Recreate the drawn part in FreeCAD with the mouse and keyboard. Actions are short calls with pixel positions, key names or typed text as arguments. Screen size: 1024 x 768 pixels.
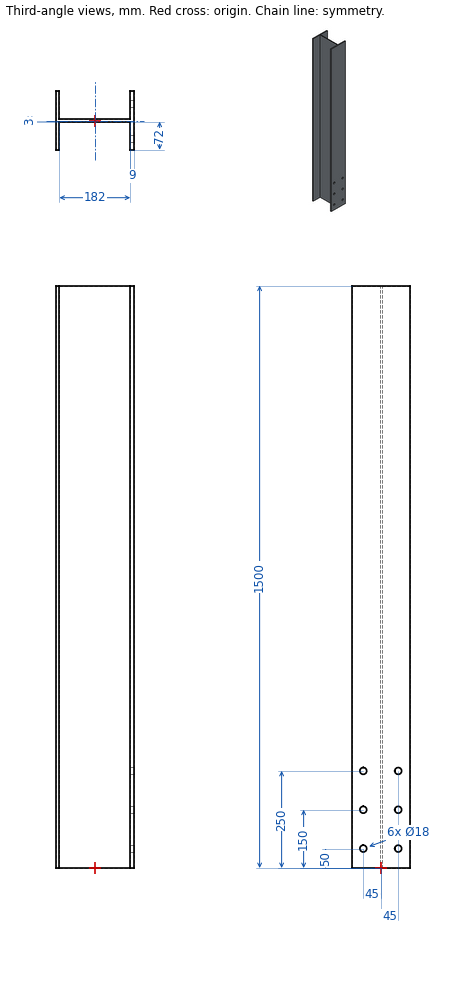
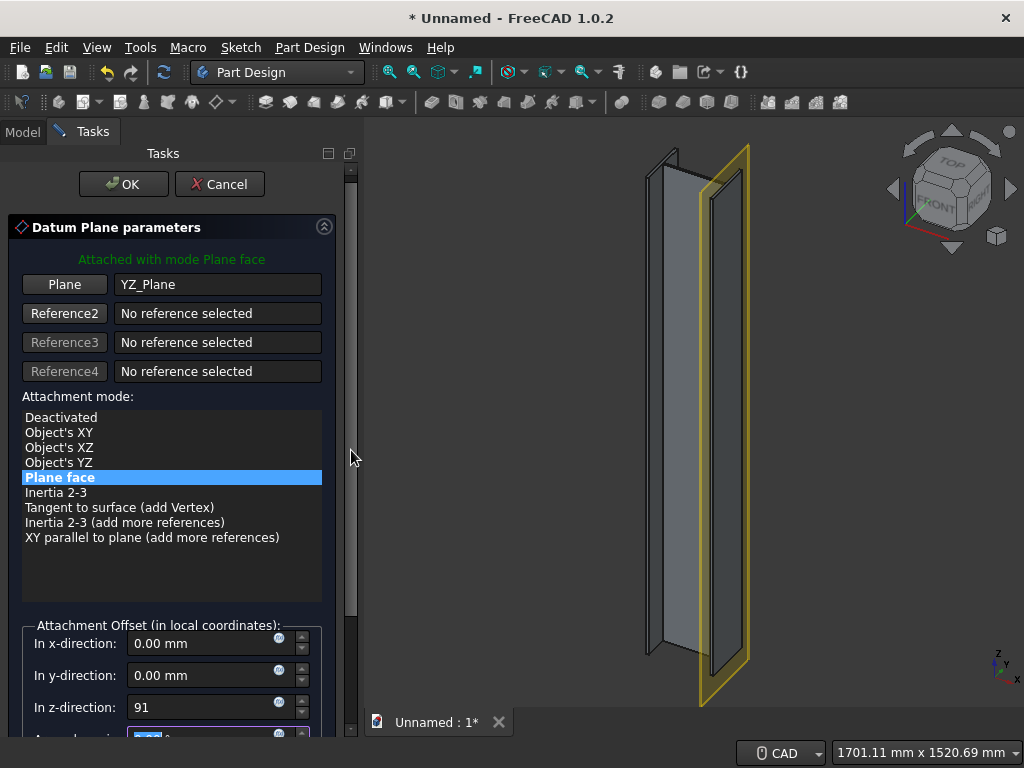
click(124, 192)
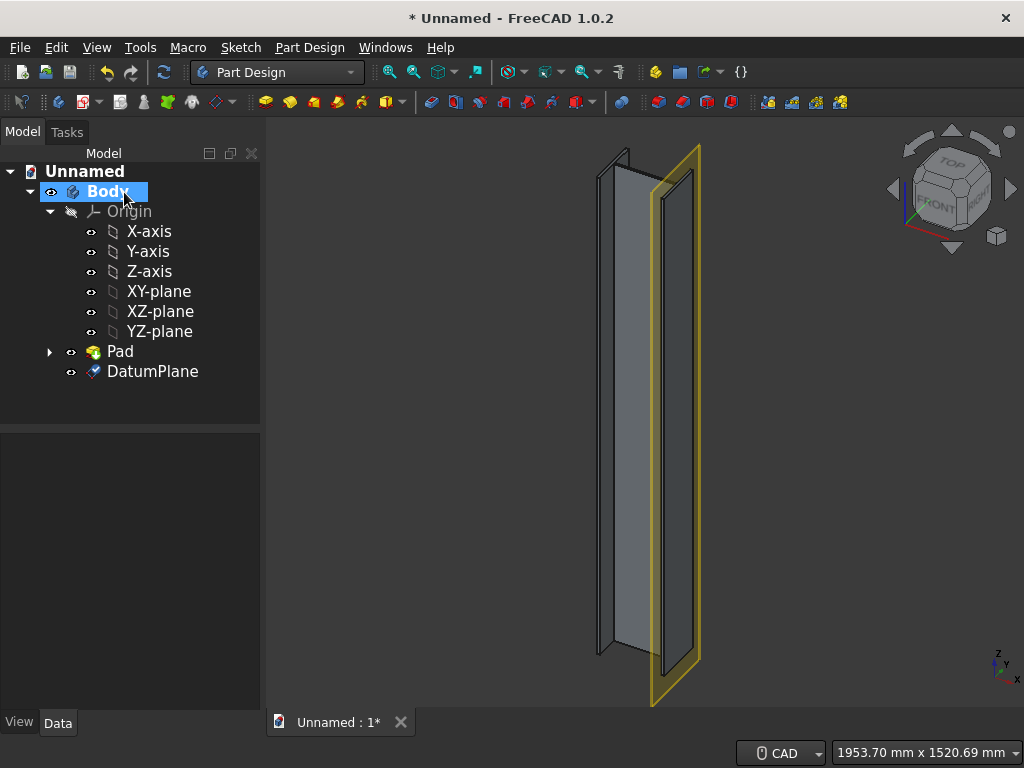
click(116, 372)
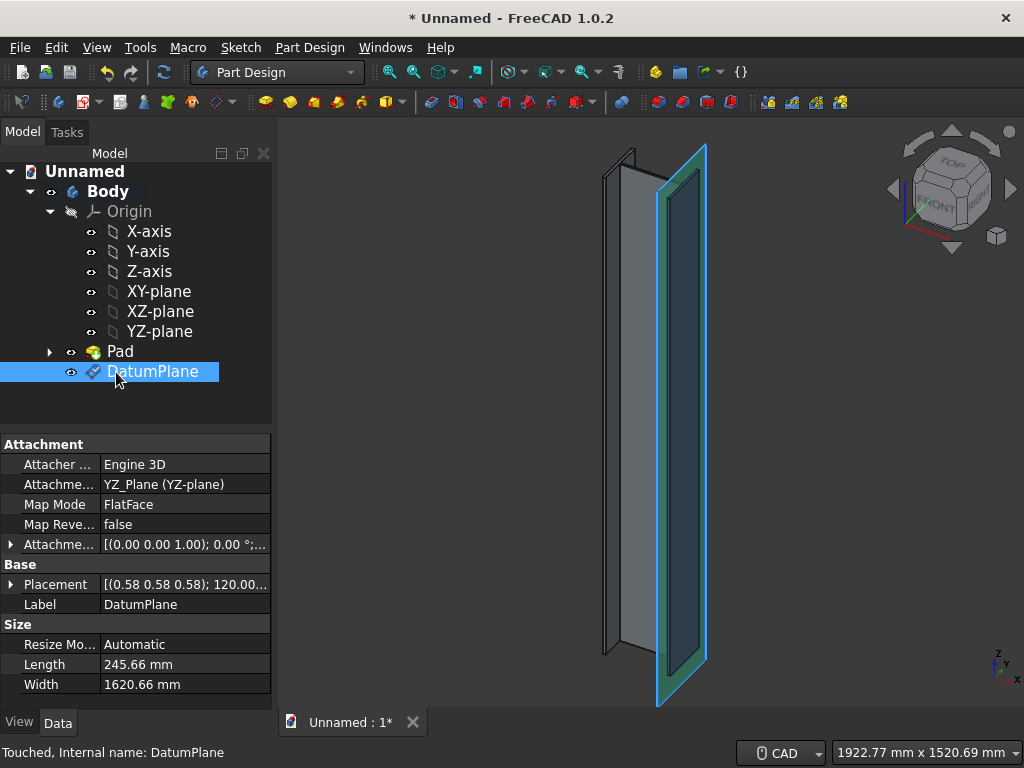
click(84, 102)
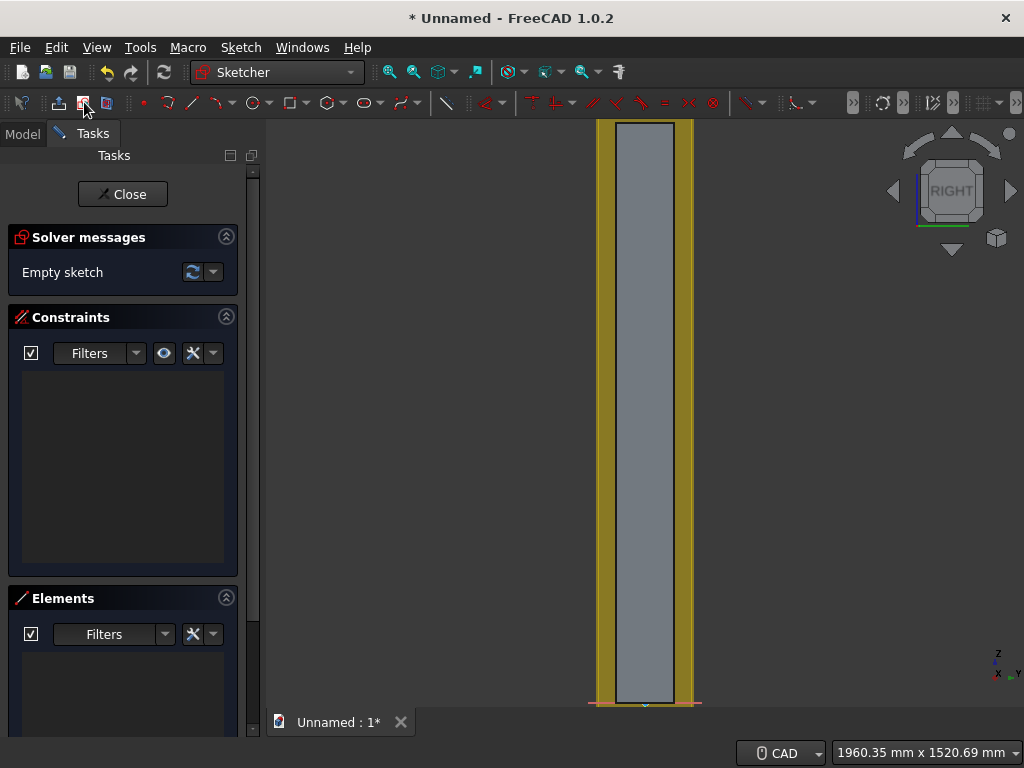
click(108, 104)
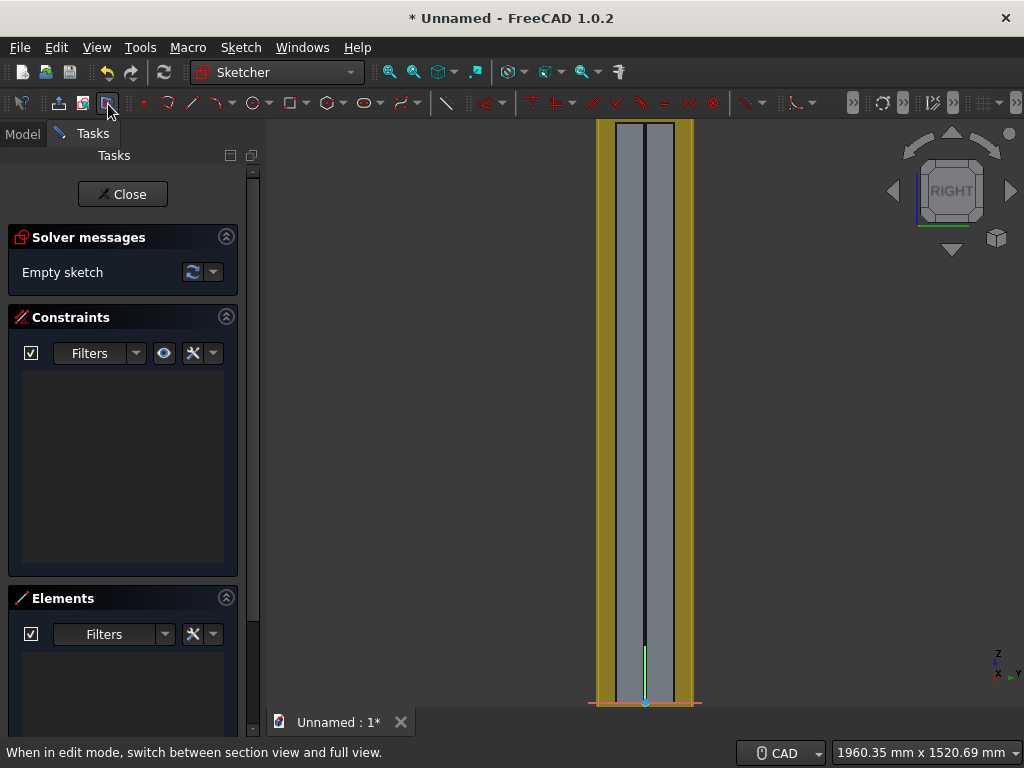
scroll(576, 413, down, 5)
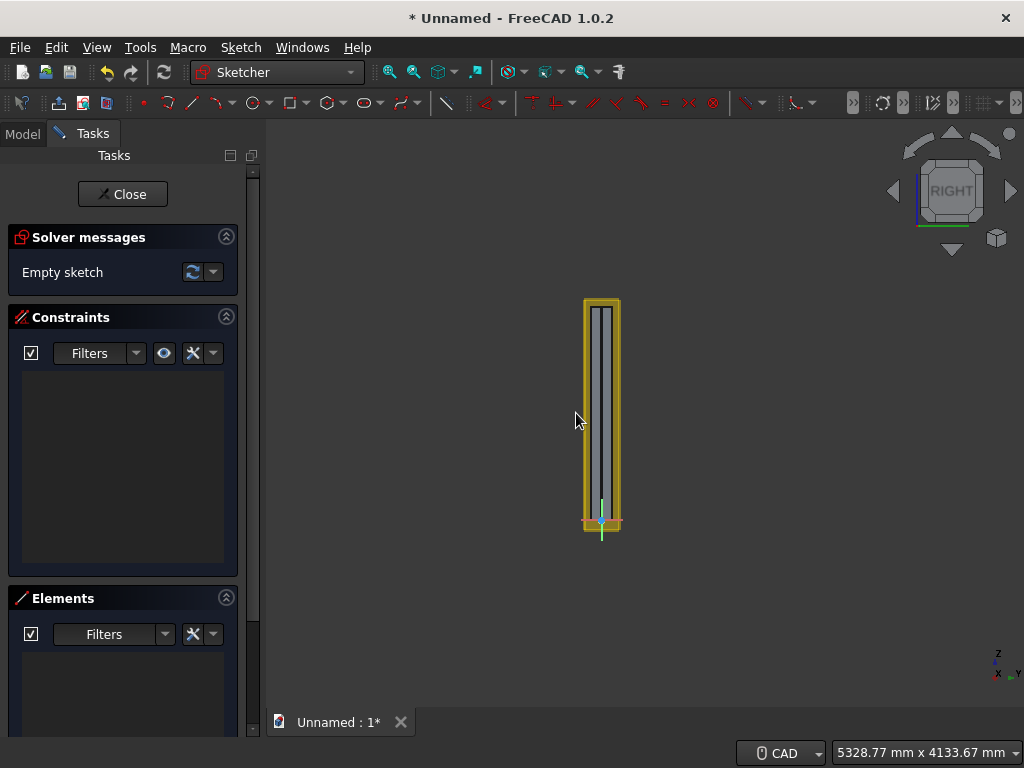
scroll(604, 510, up, 12)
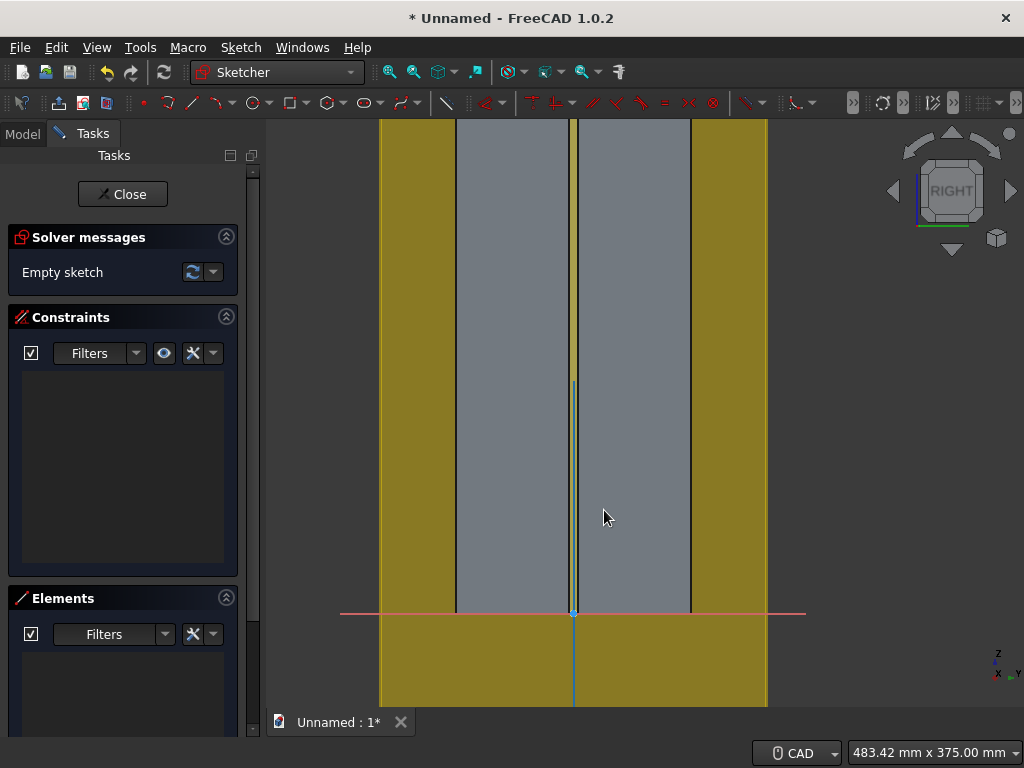
click(254, 104)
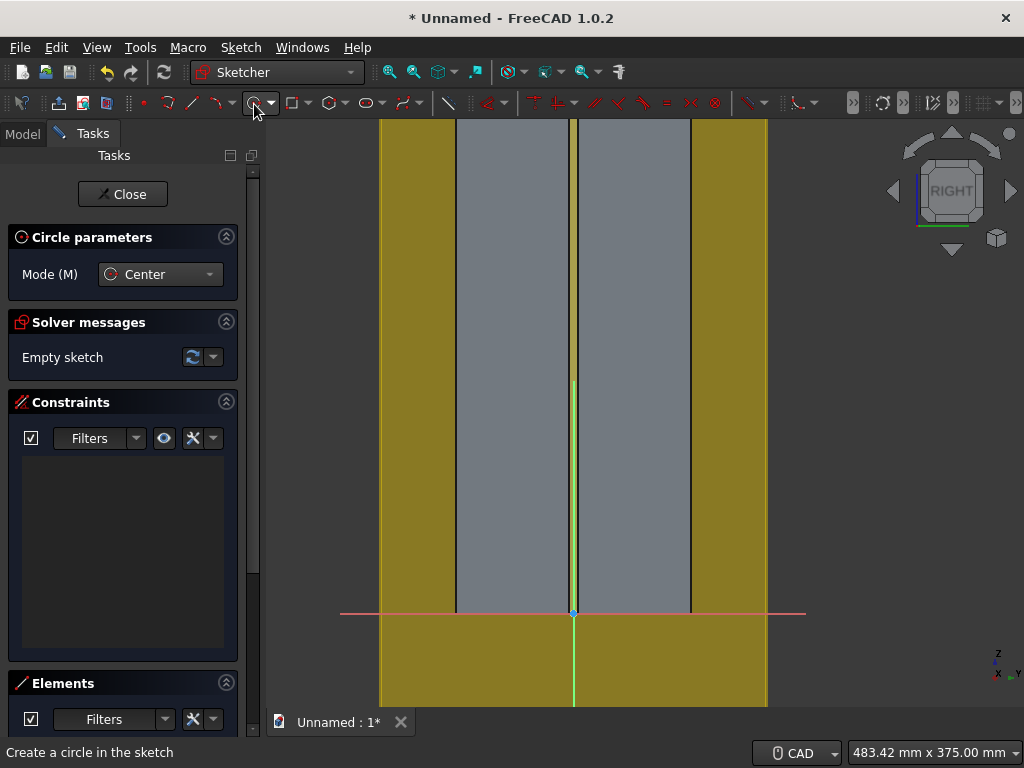
scroll(503, 535, up, 3)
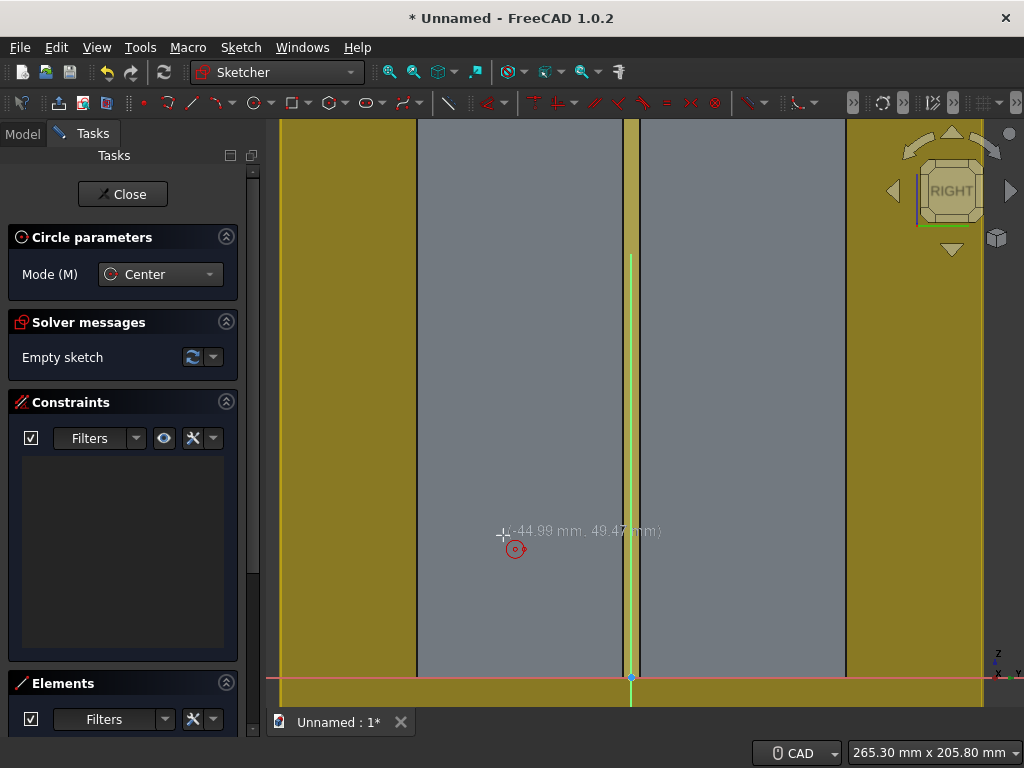
click(503, 535)
click(521, 517)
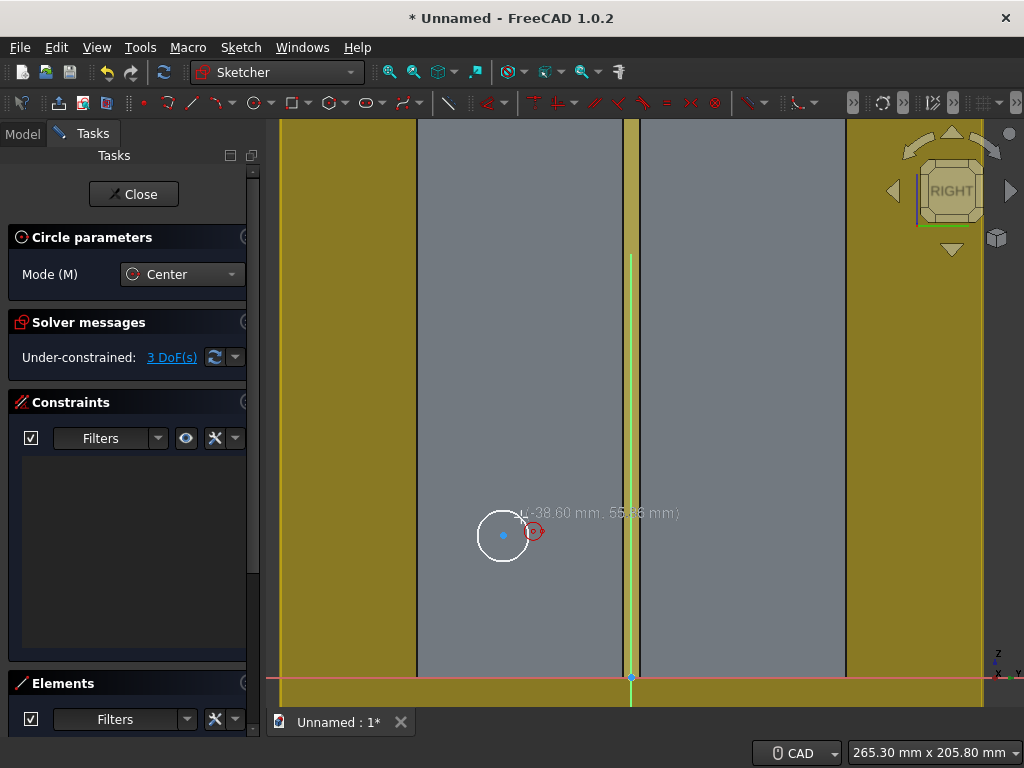
click(503, 249)
click(521, 231)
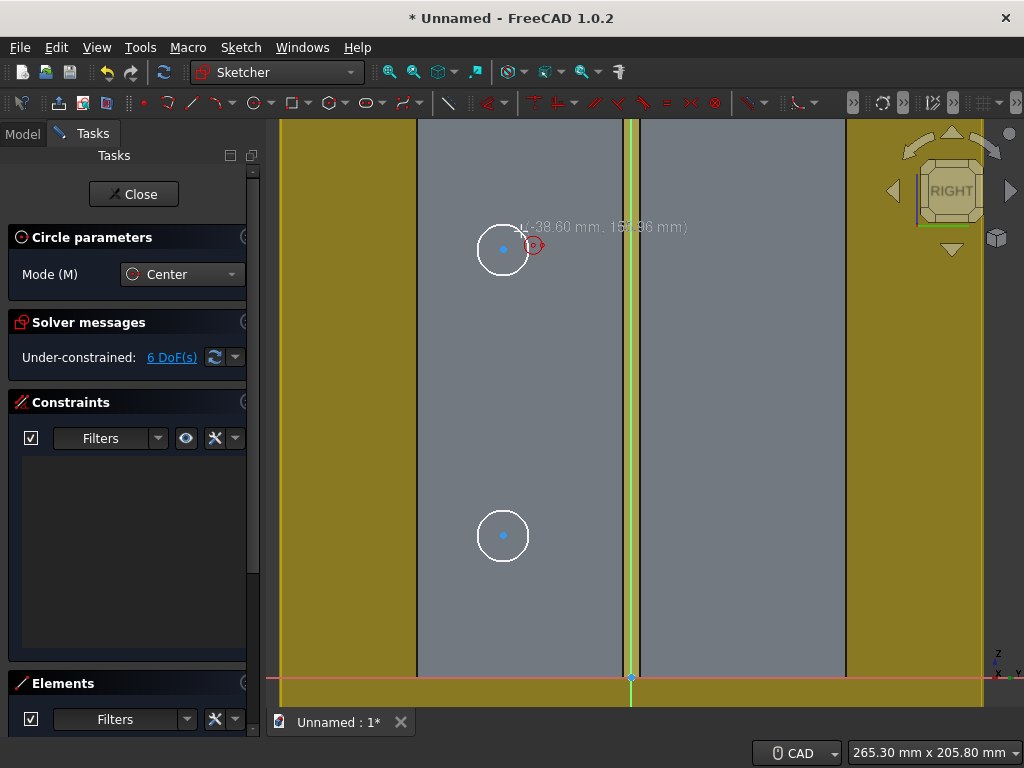
scroll(510, 541, down, 3)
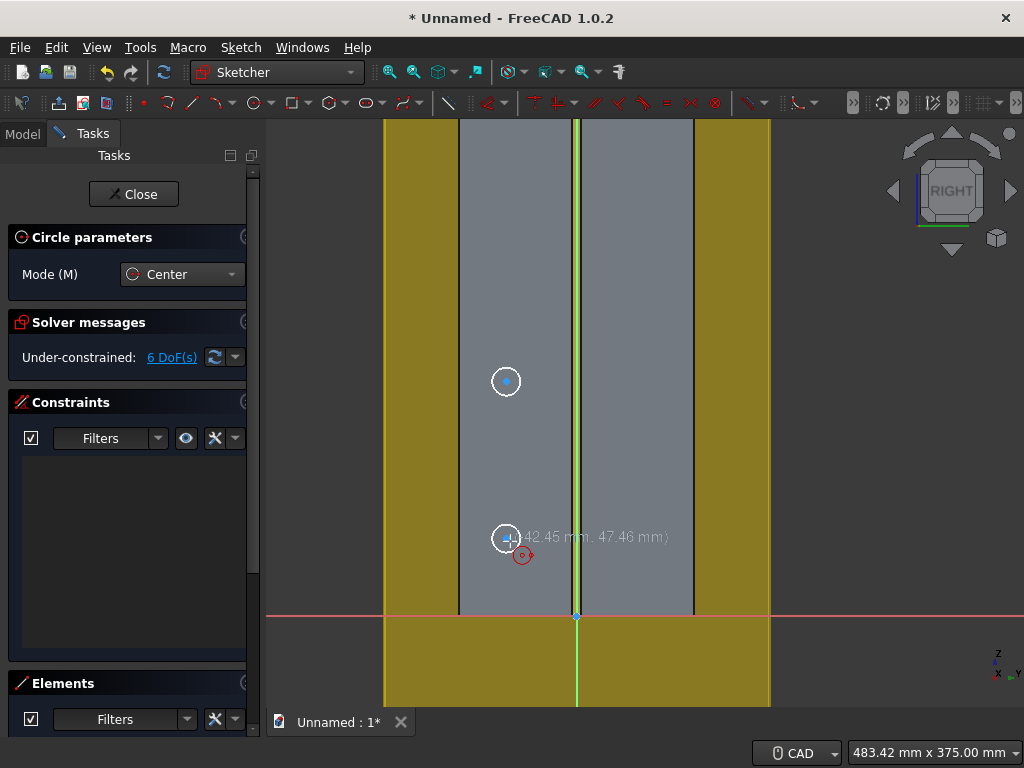
scroll(506, 224, up, 3)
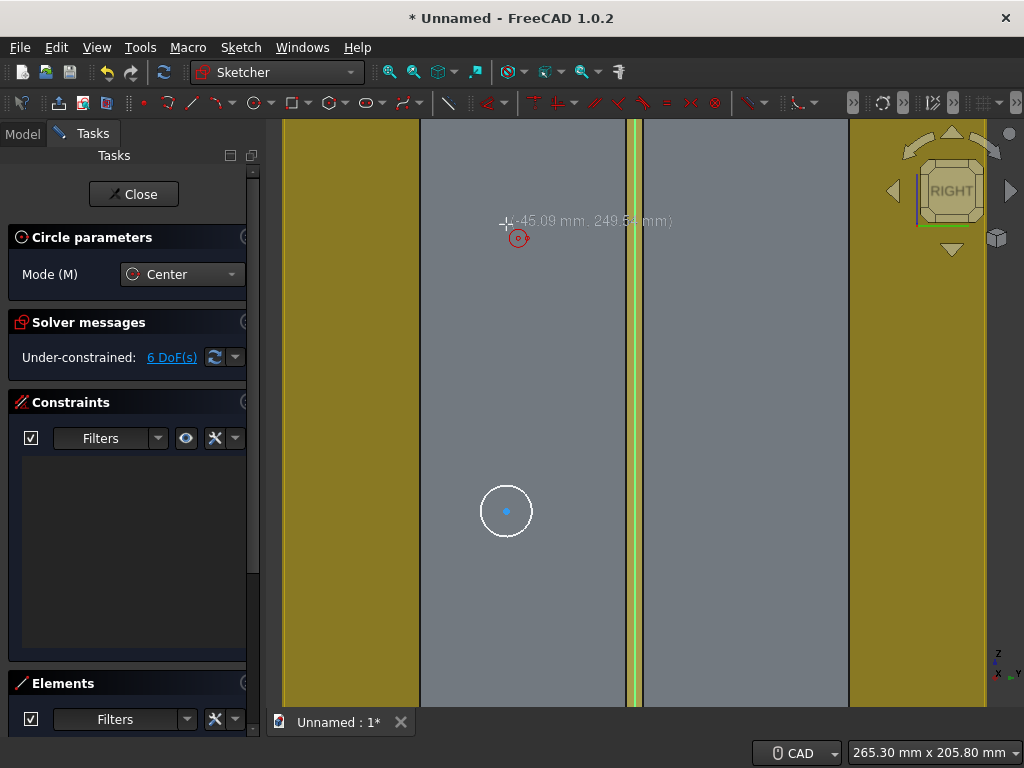
click(506, 224)
click(524, 206)